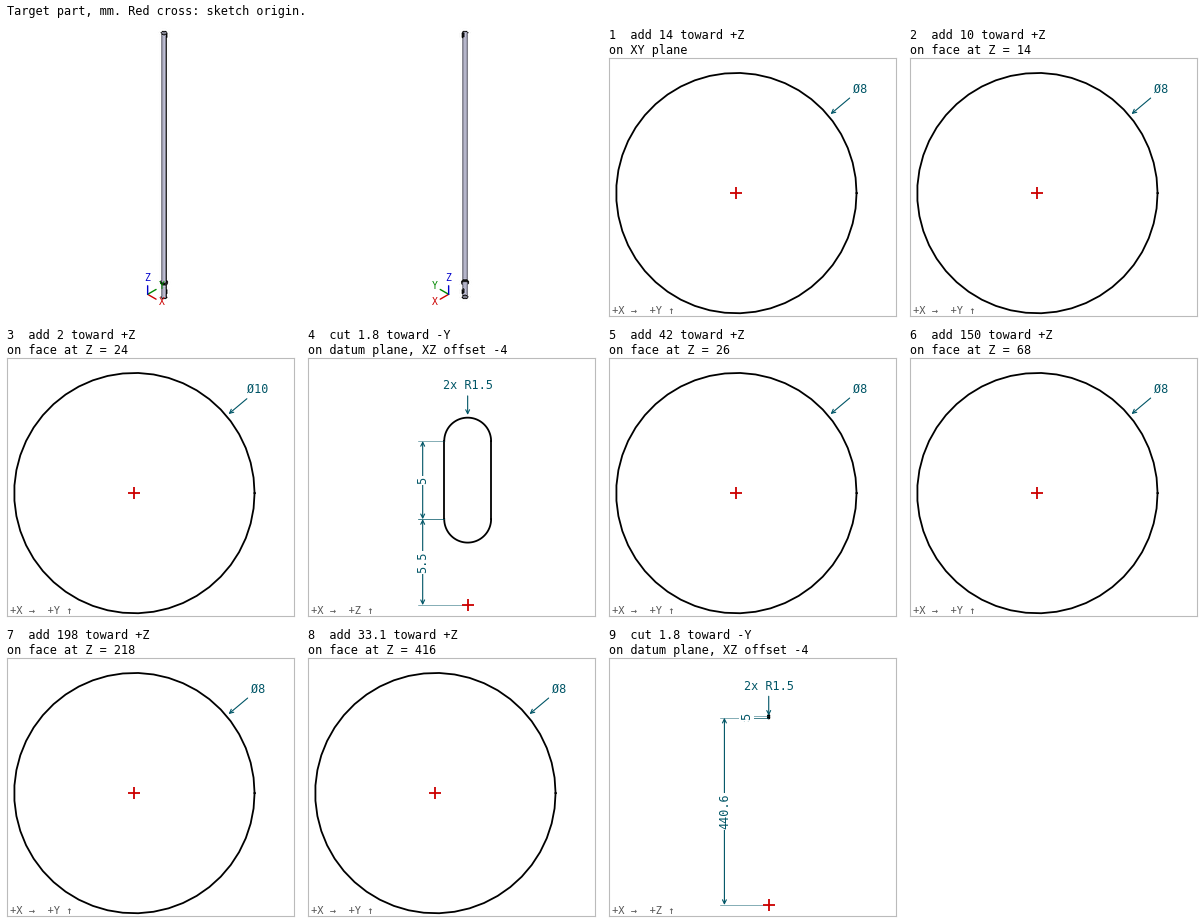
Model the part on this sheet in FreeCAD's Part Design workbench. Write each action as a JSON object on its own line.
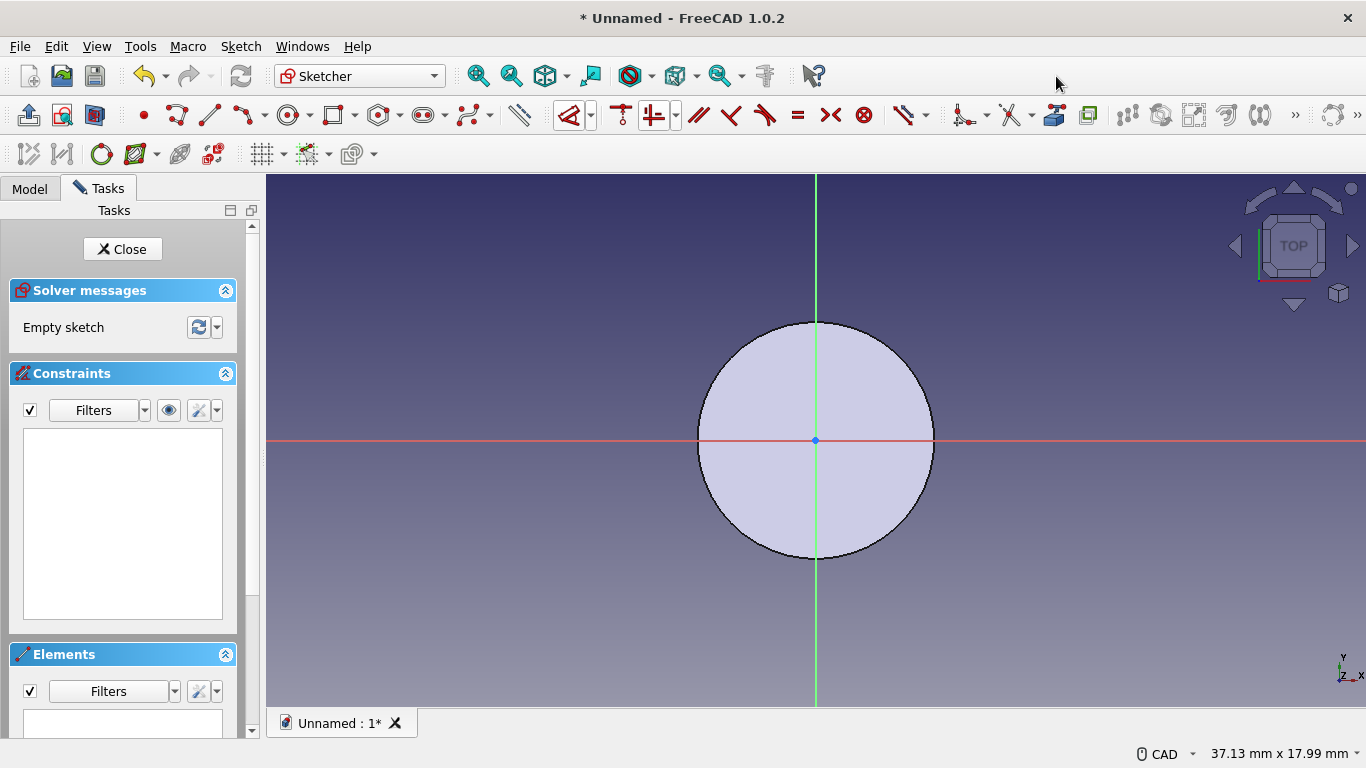
{"action": "scroll", "coordinate": [955, 440], "scroll_direction": "up", "scroll_amount": 2}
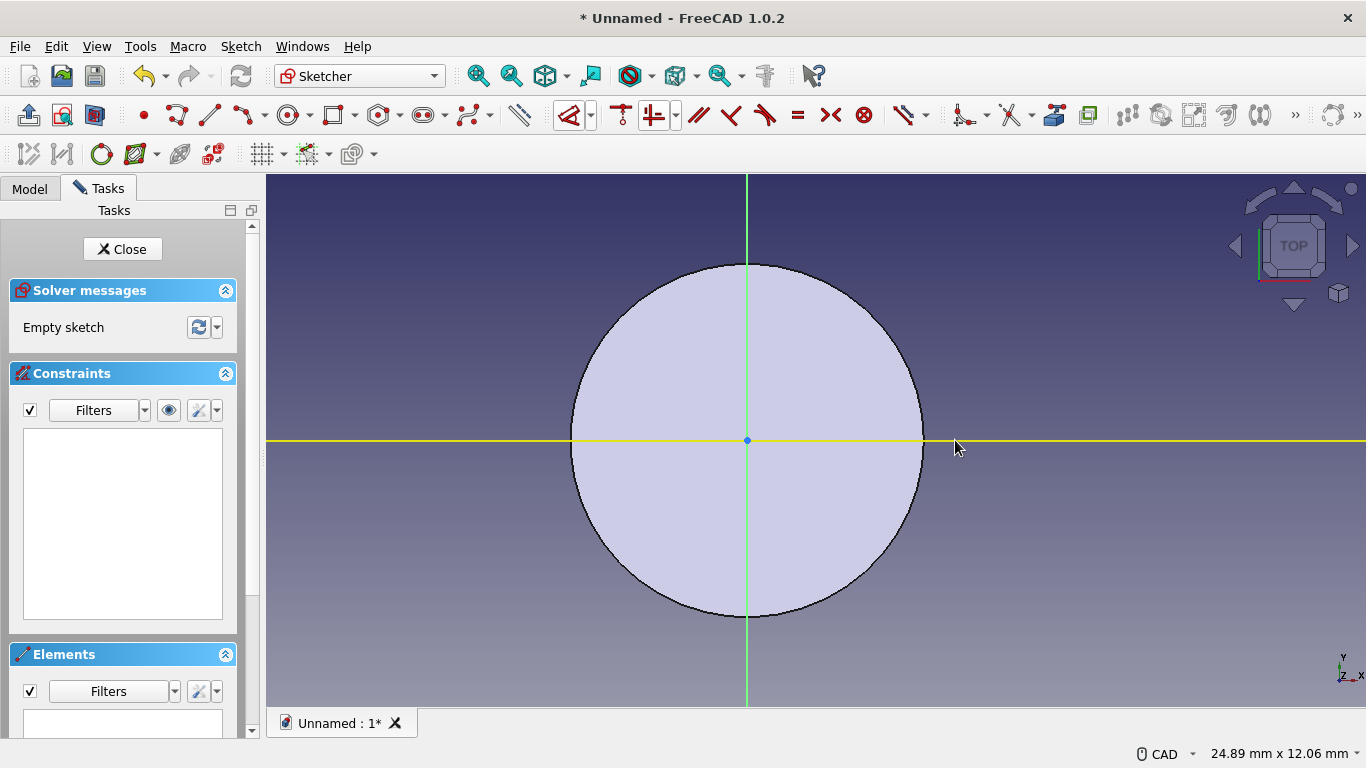
{"action": "left_click", "coordinate": [288, 116]}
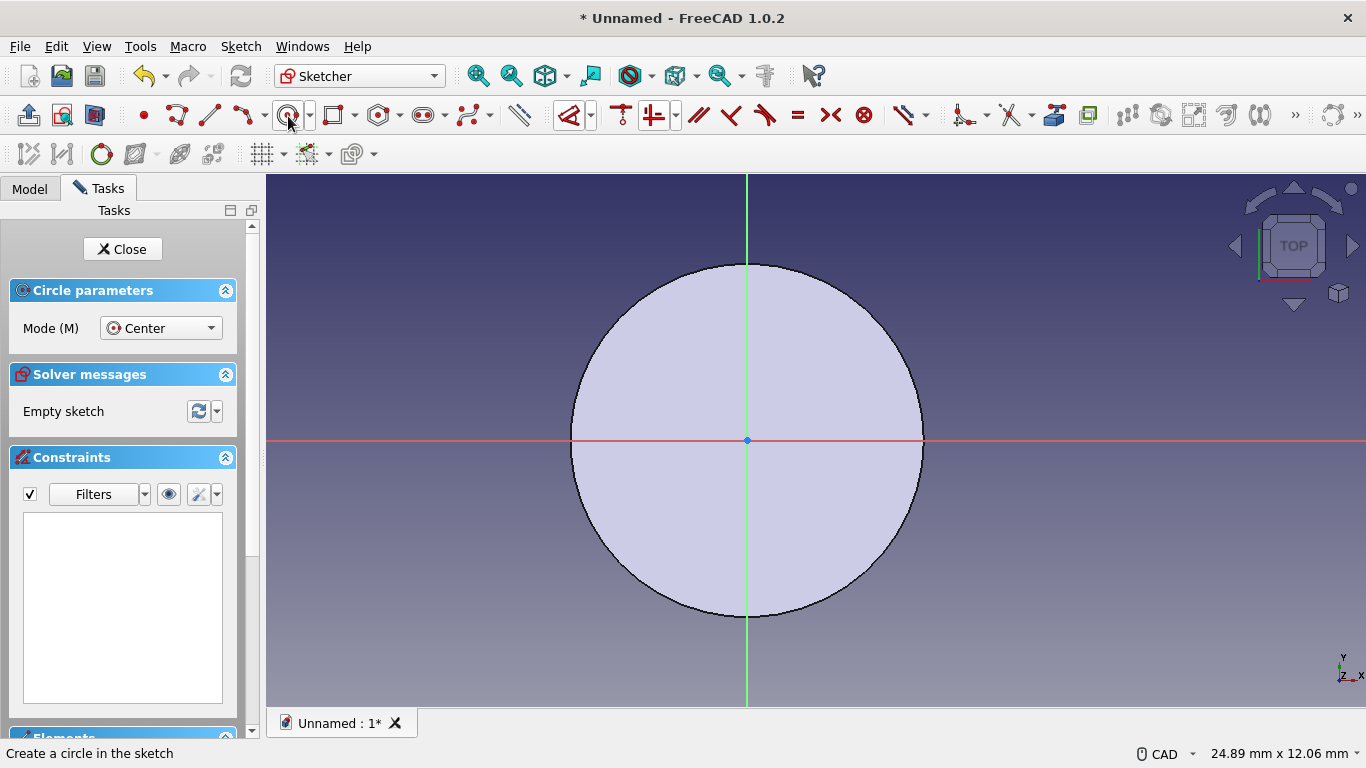
{"action": "left_click", "coordinate": [747, 440]}
{"action": "left_click", "coordinate": [872, 316]}
{"action": "key", "text": "Escape"}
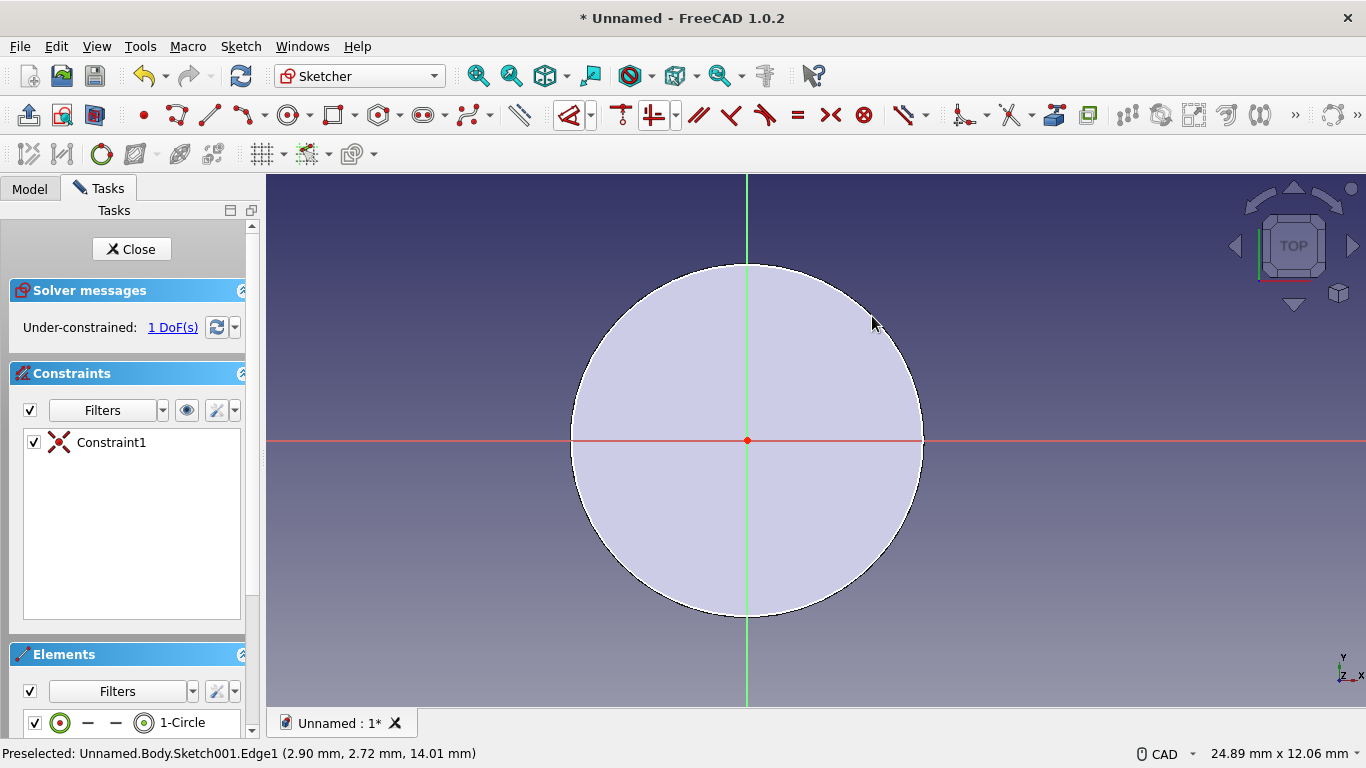
{"action": "left_click", "coordinate": [871, 316]}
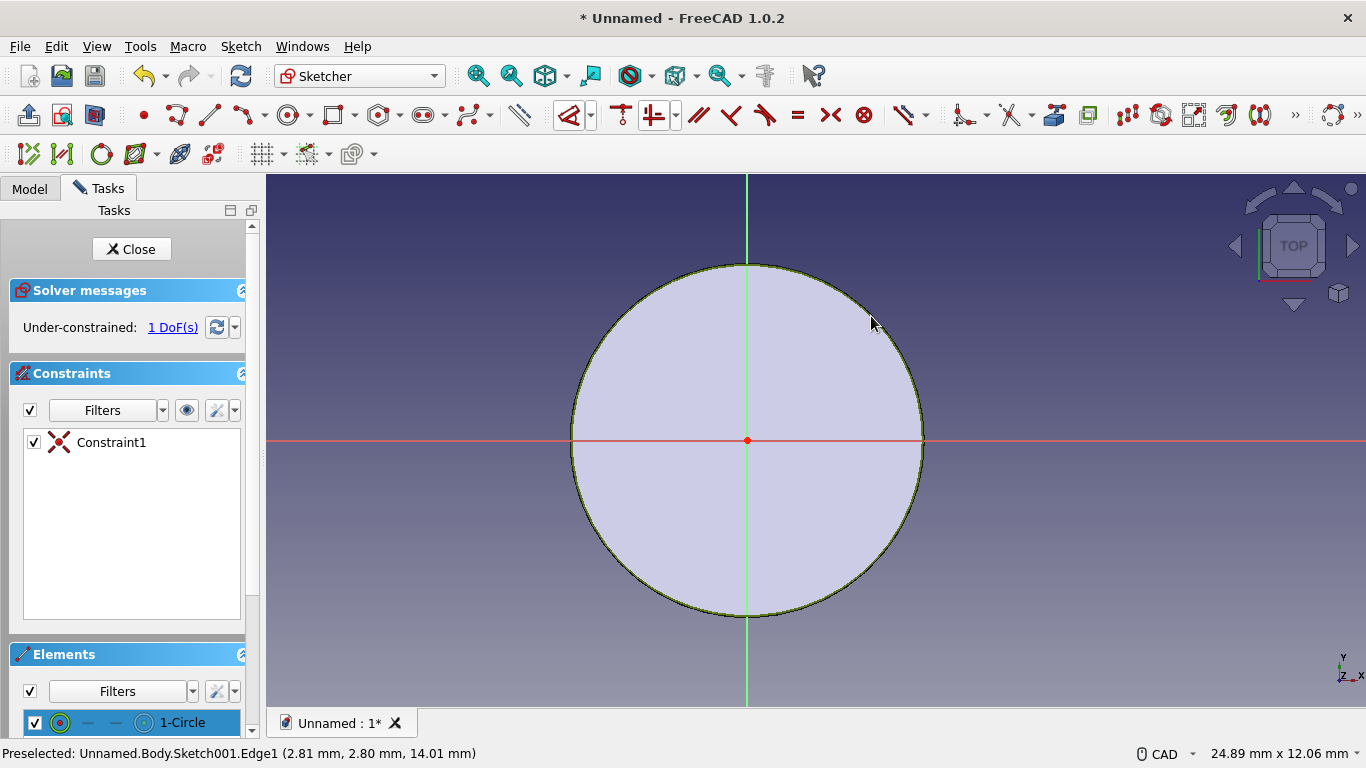
{"action": "key", "text": "k o"}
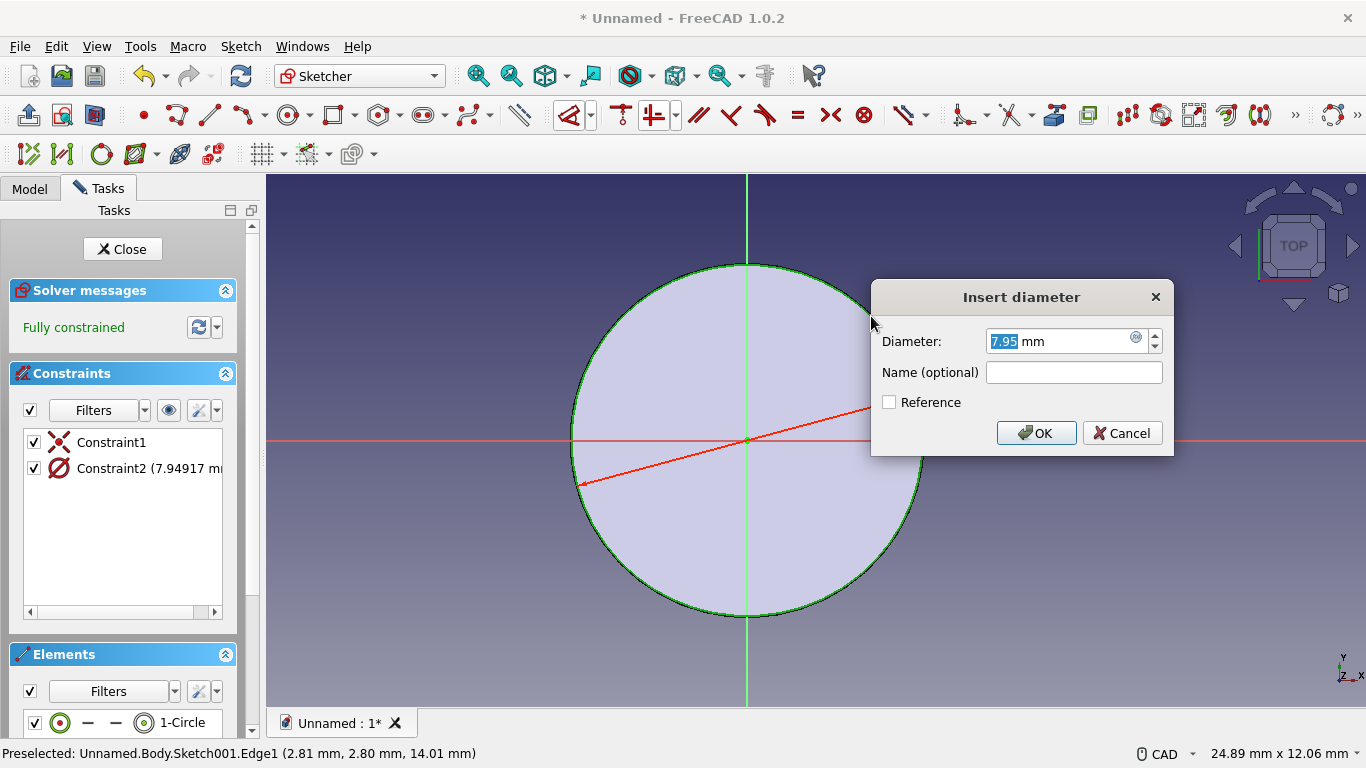
{"action": "type", "text": "8"}
{"action": "key", "text": "Return"}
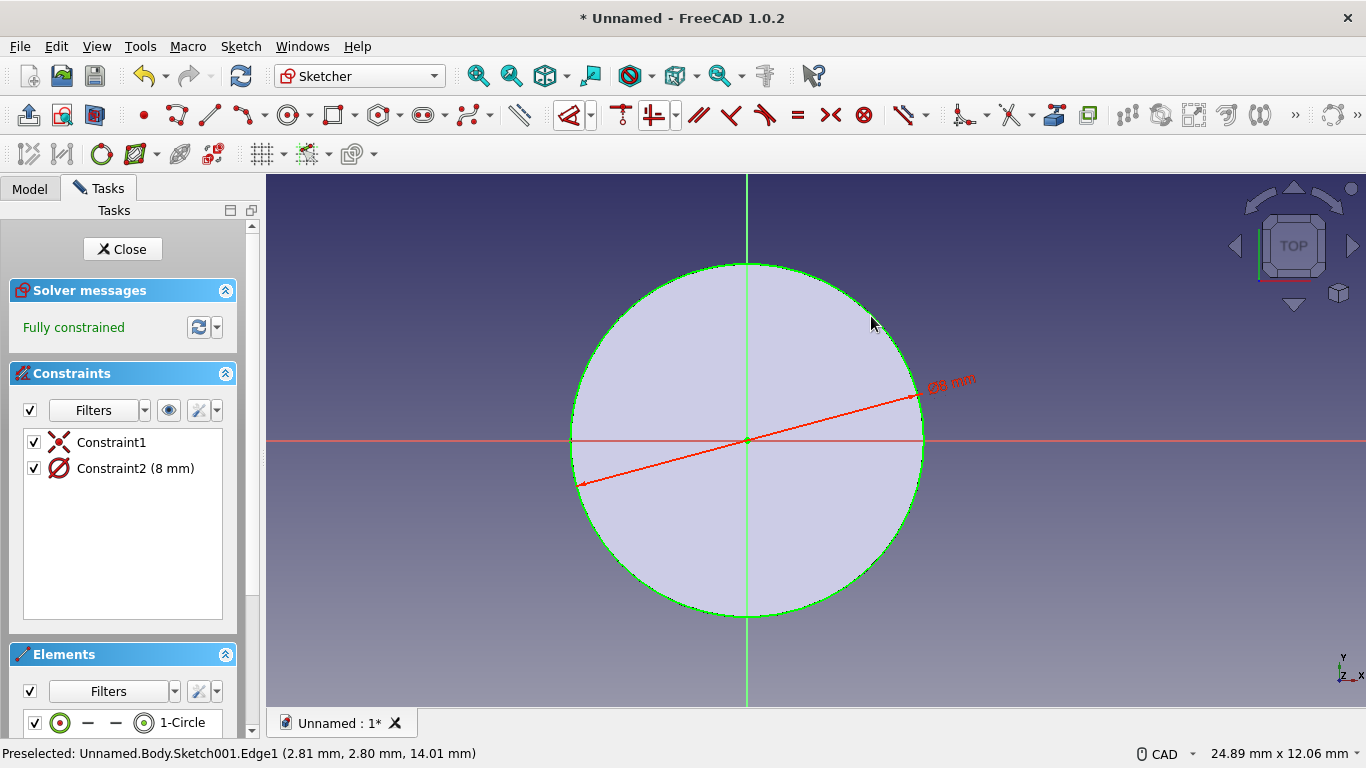
{"action": "left_click", "coordinate": [123, 249]}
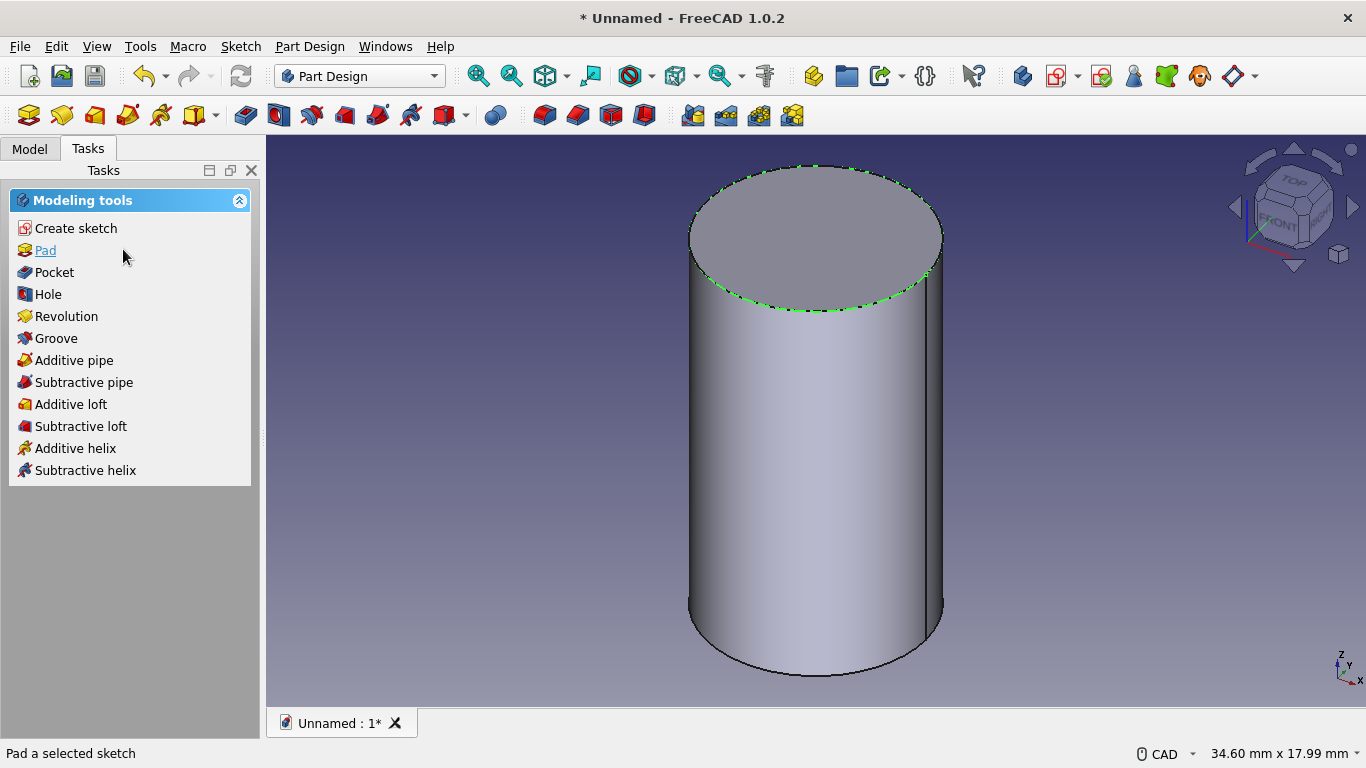
{"action": "left_click", "coordinate": [29, 116]}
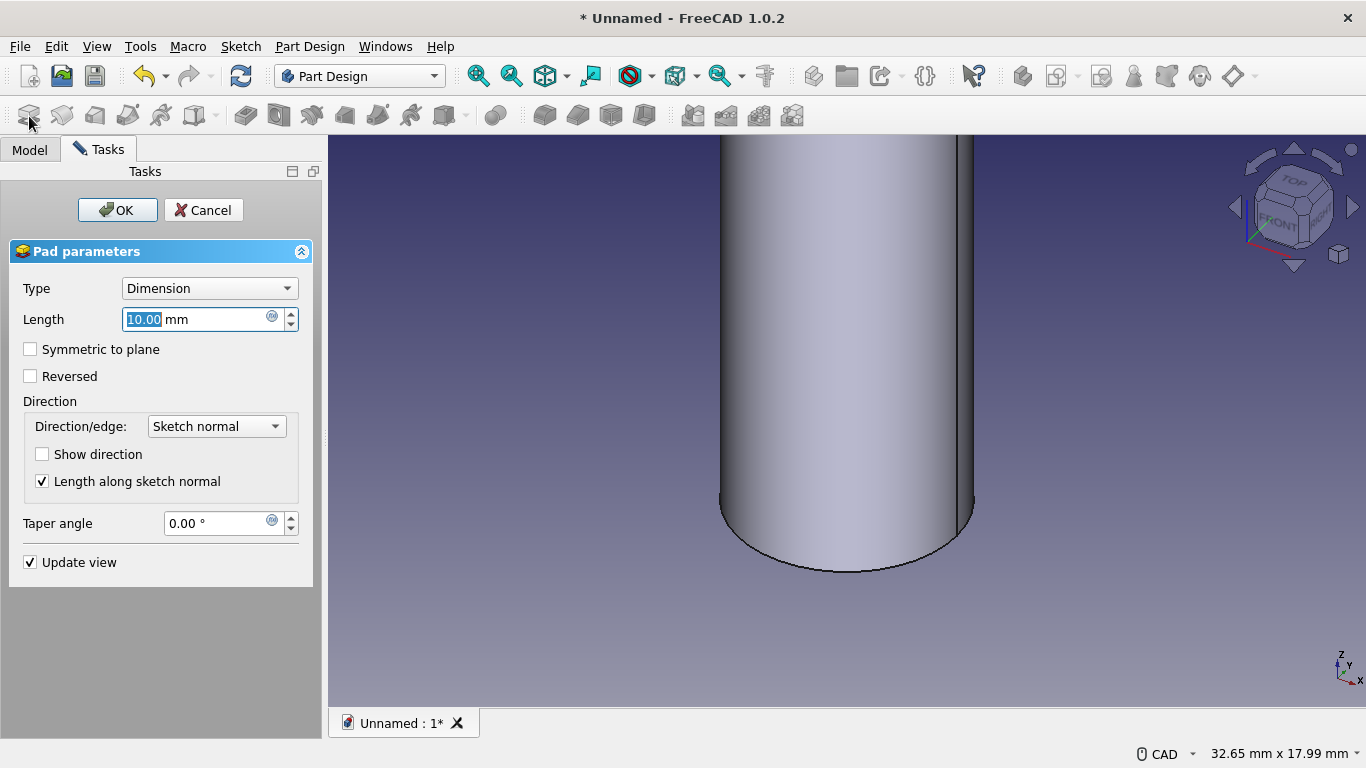
{"action": "type", "text": "10"}
{"action": "key", "text": "Tab"}